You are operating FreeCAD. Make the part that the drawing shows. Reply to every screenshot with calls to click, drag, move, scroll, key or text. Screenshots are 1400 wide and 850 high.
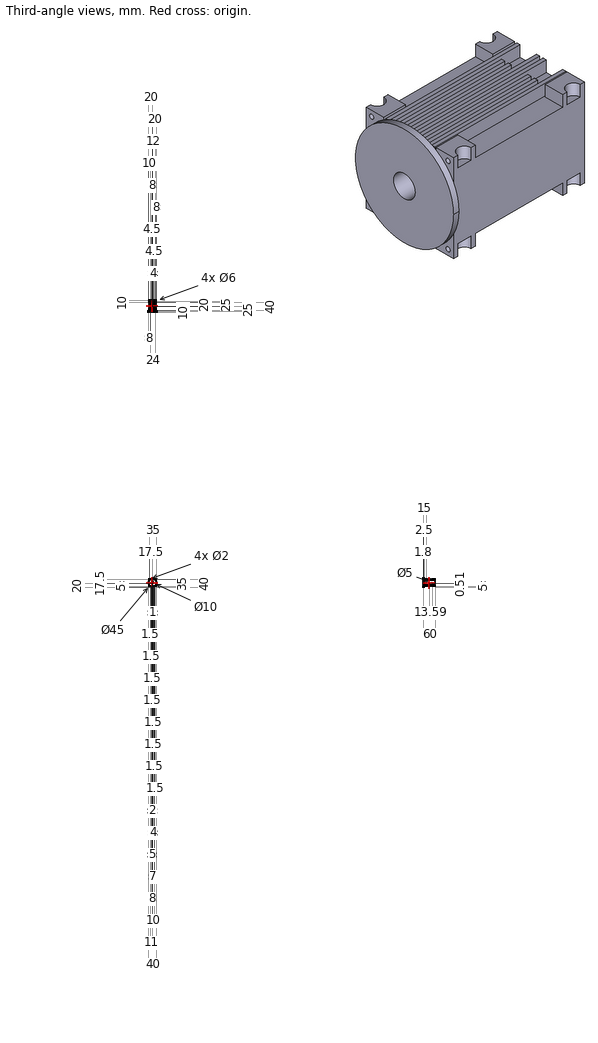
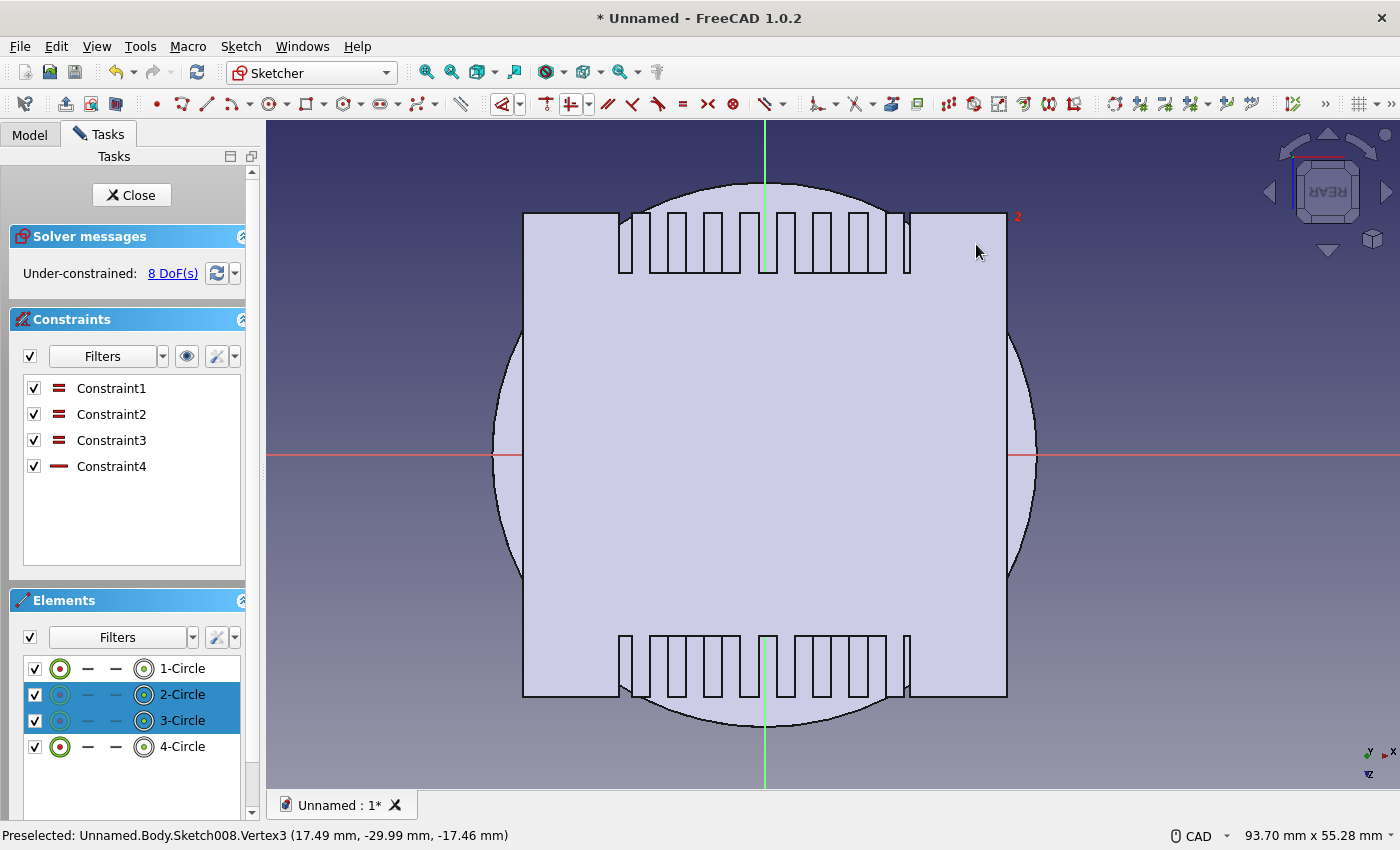
key(v)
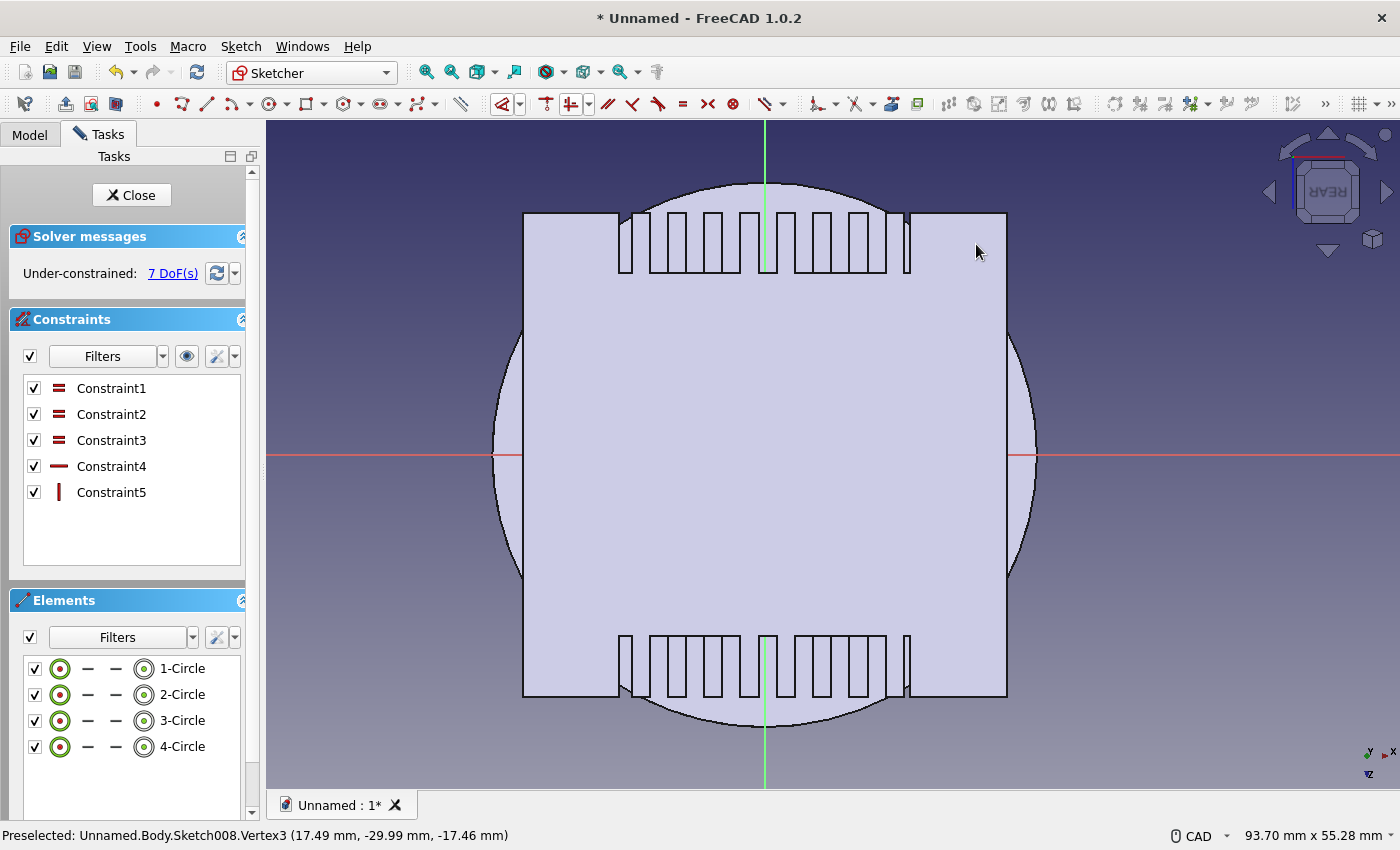
click(553, 667)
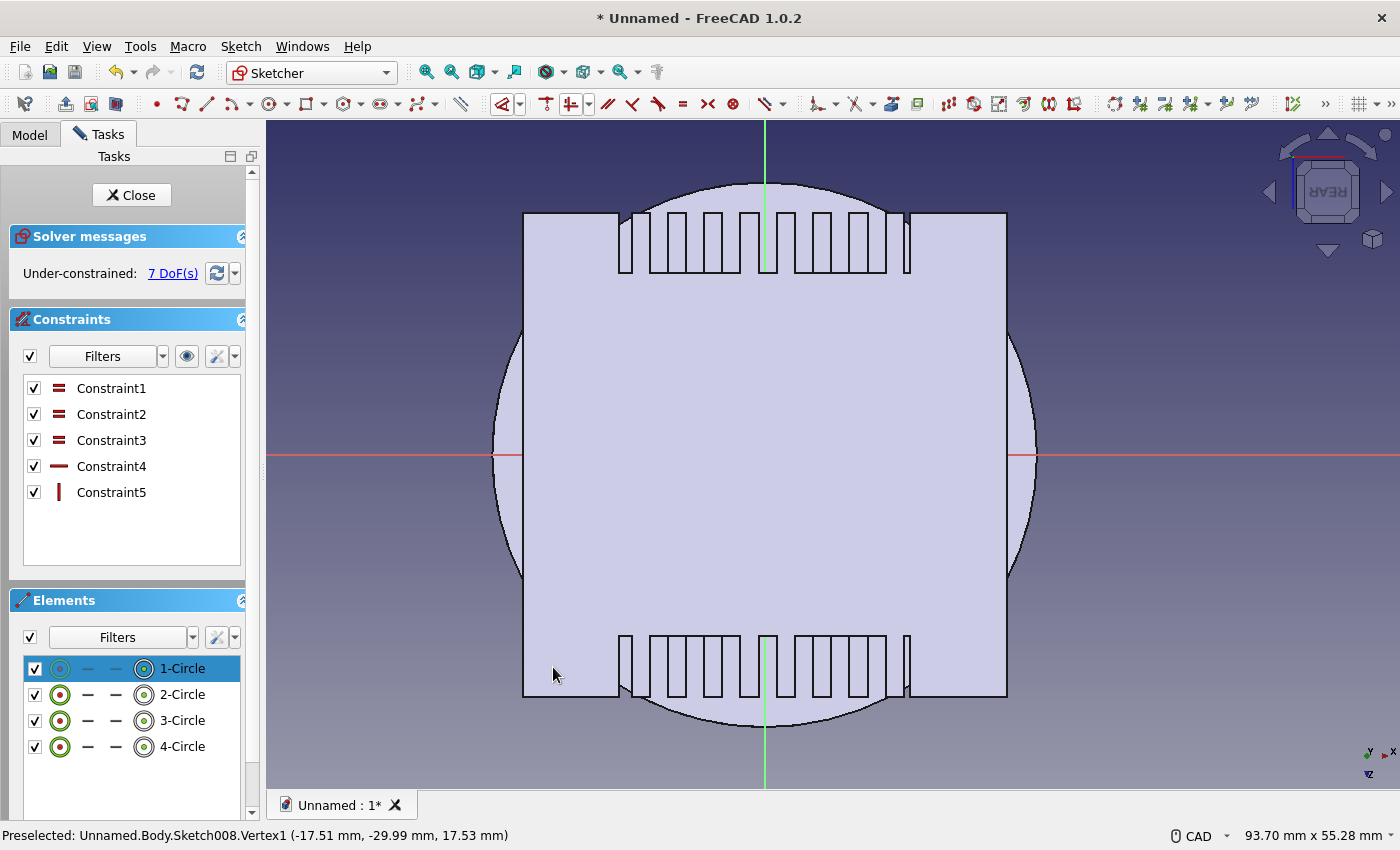
click(553, 244)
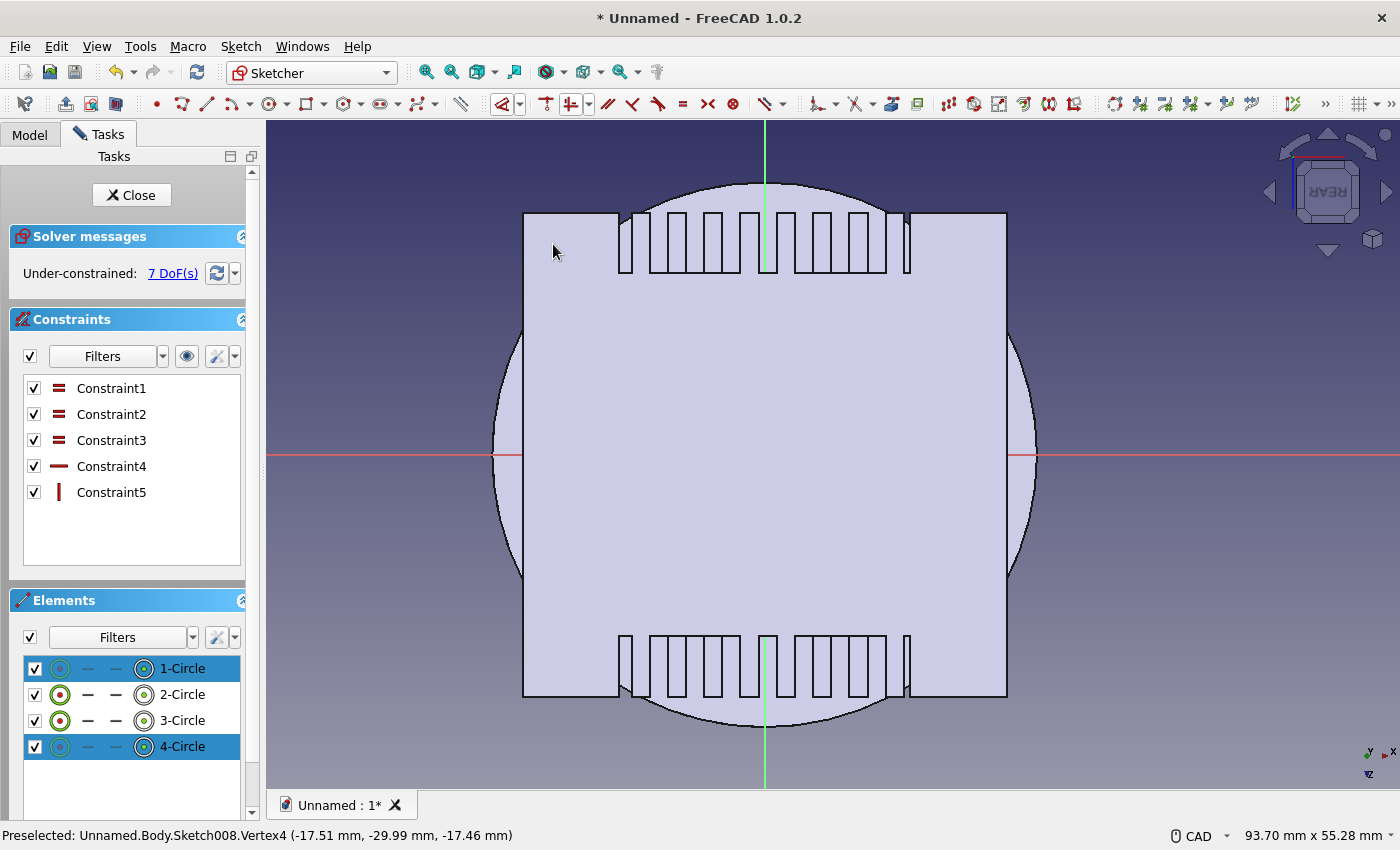
click(588, 104)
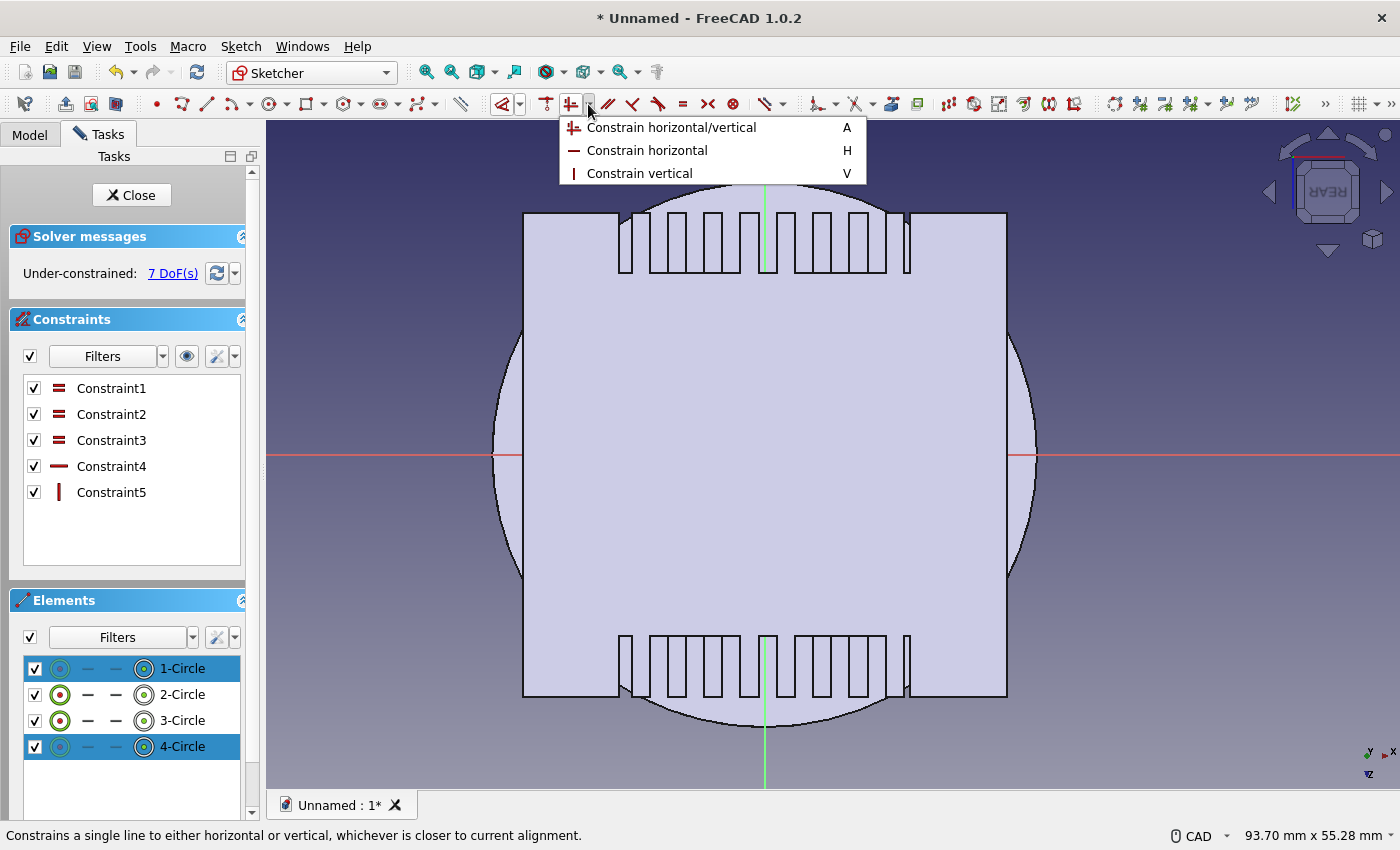
click(713, 174)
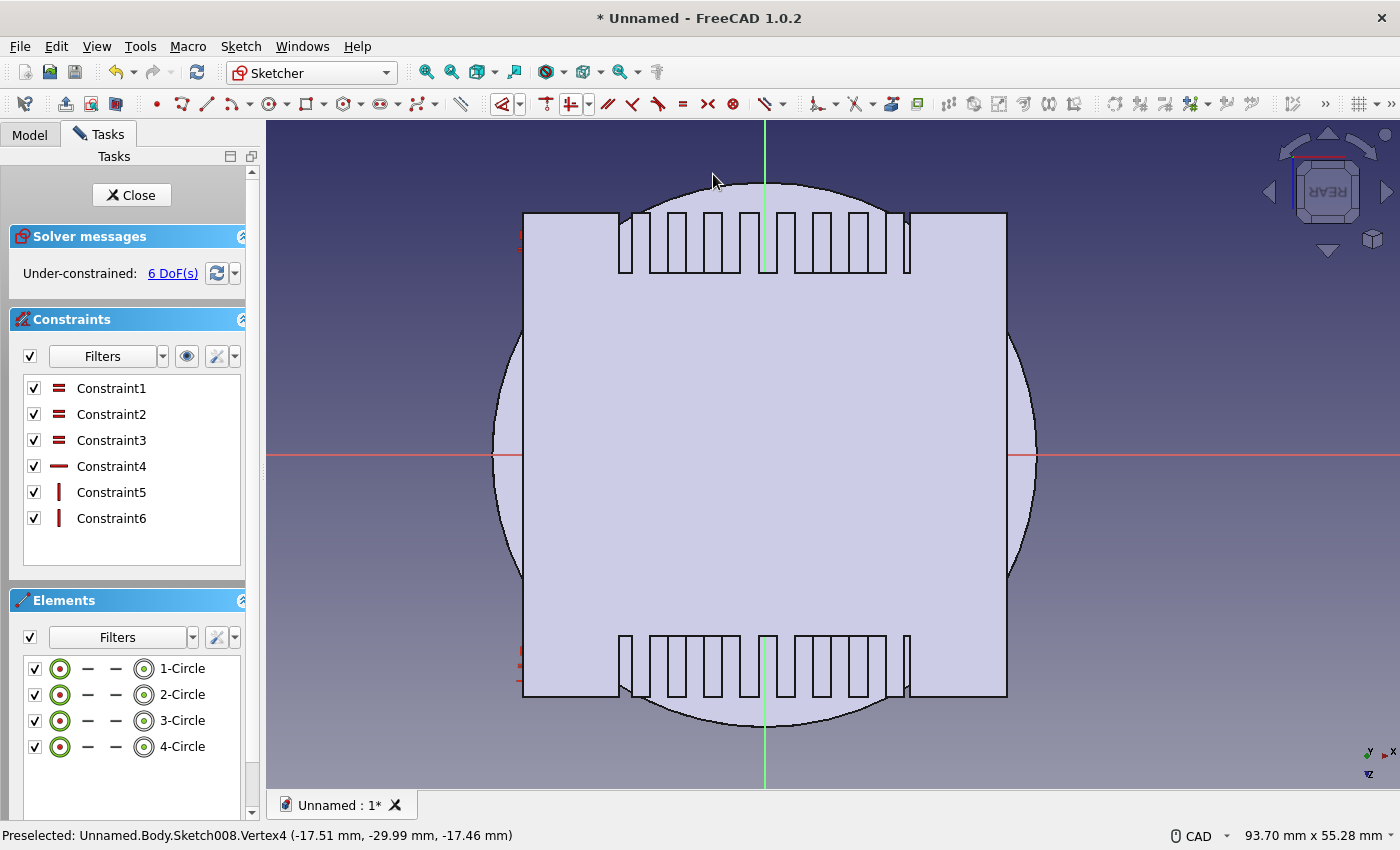
click(976, 244)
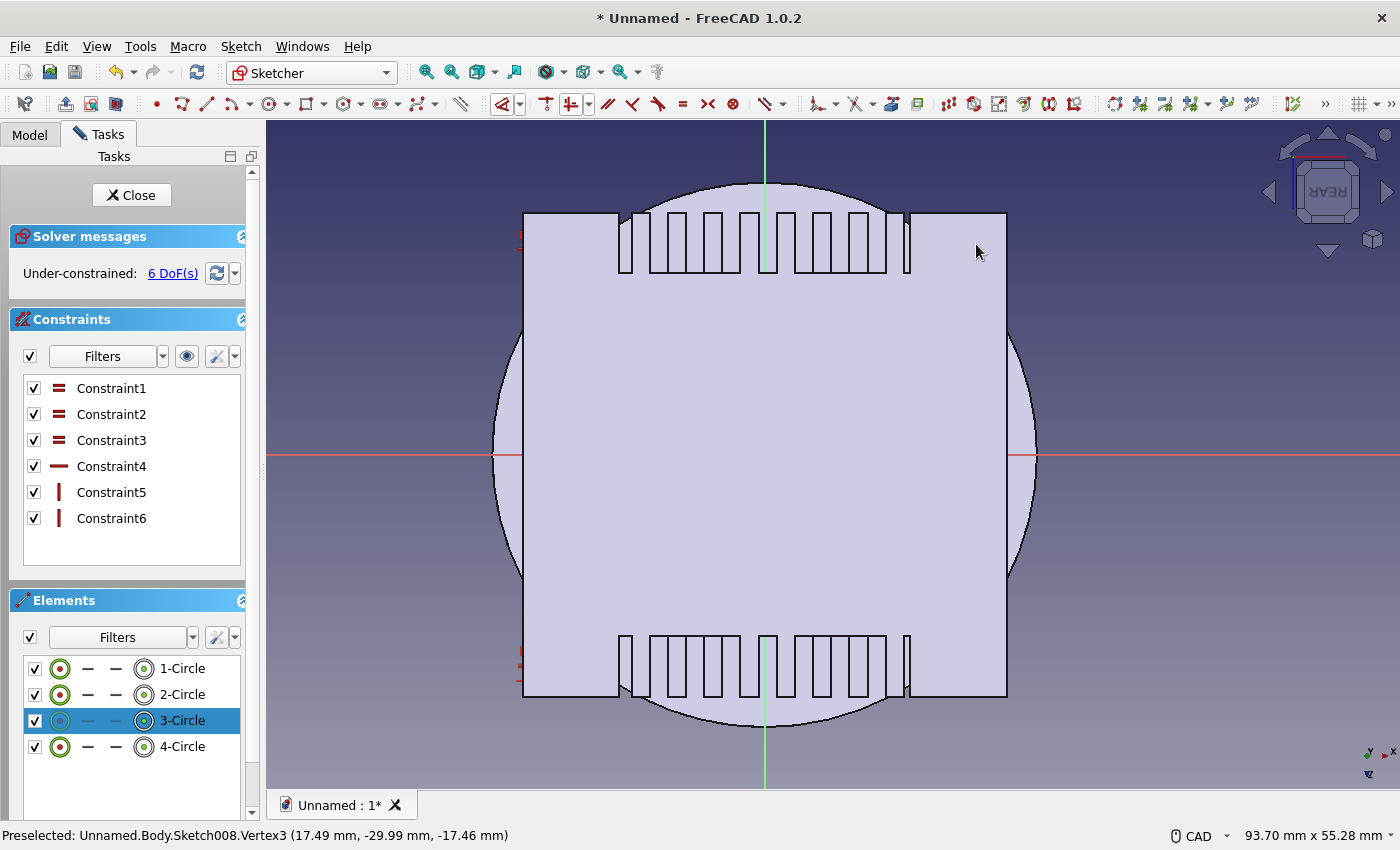
click(553, 244)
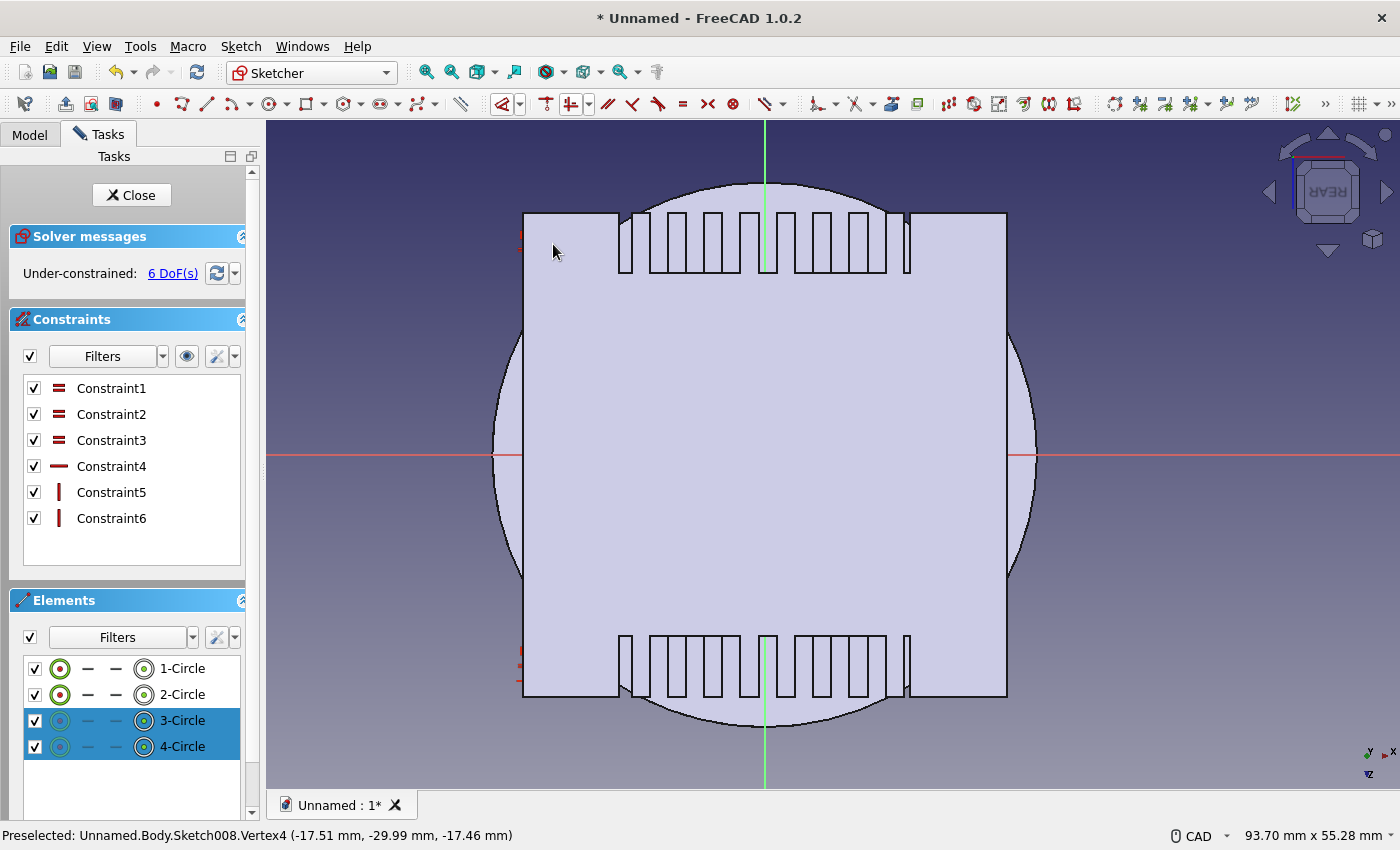
key(h)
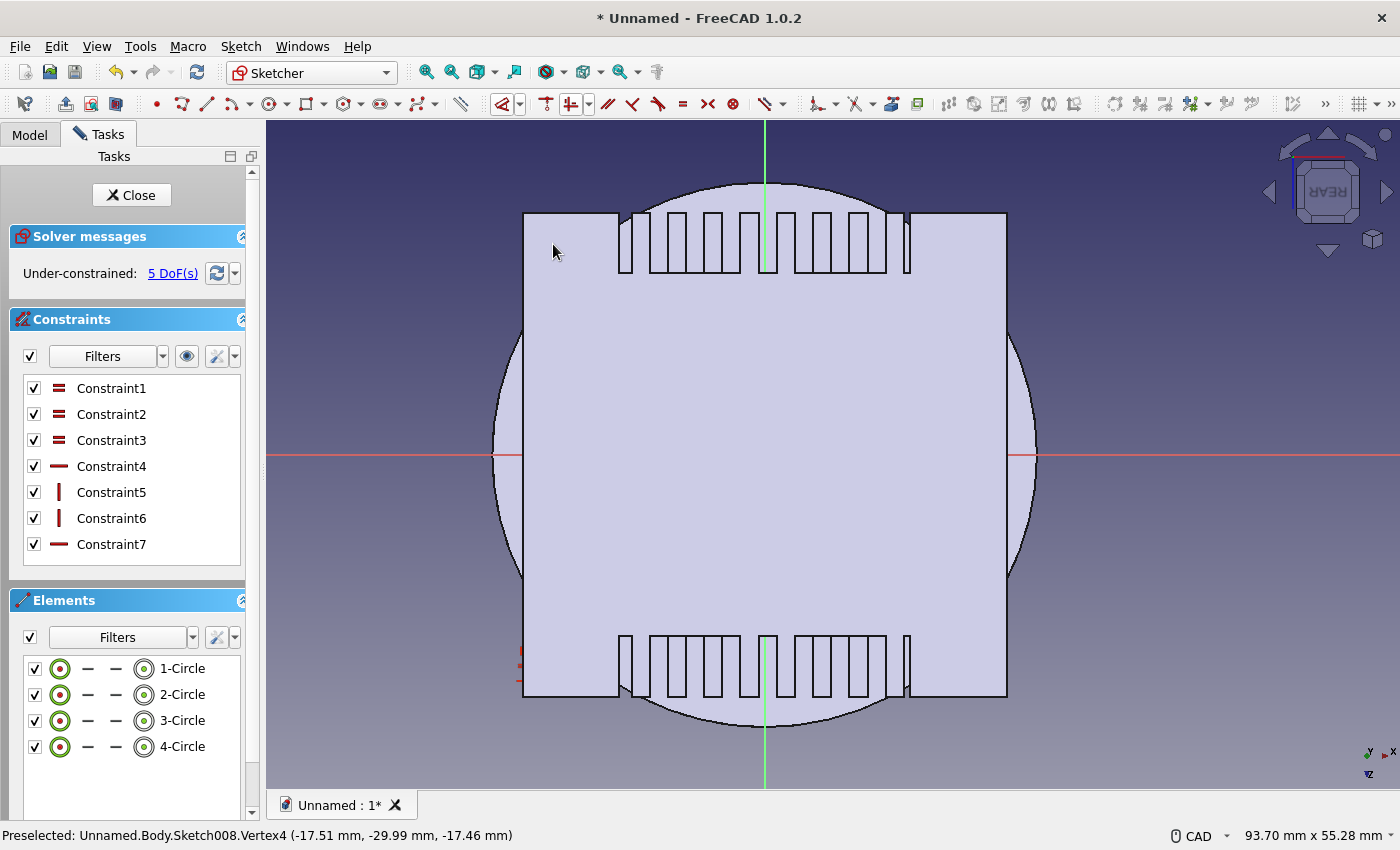
scroll(561, 658, up, 3)